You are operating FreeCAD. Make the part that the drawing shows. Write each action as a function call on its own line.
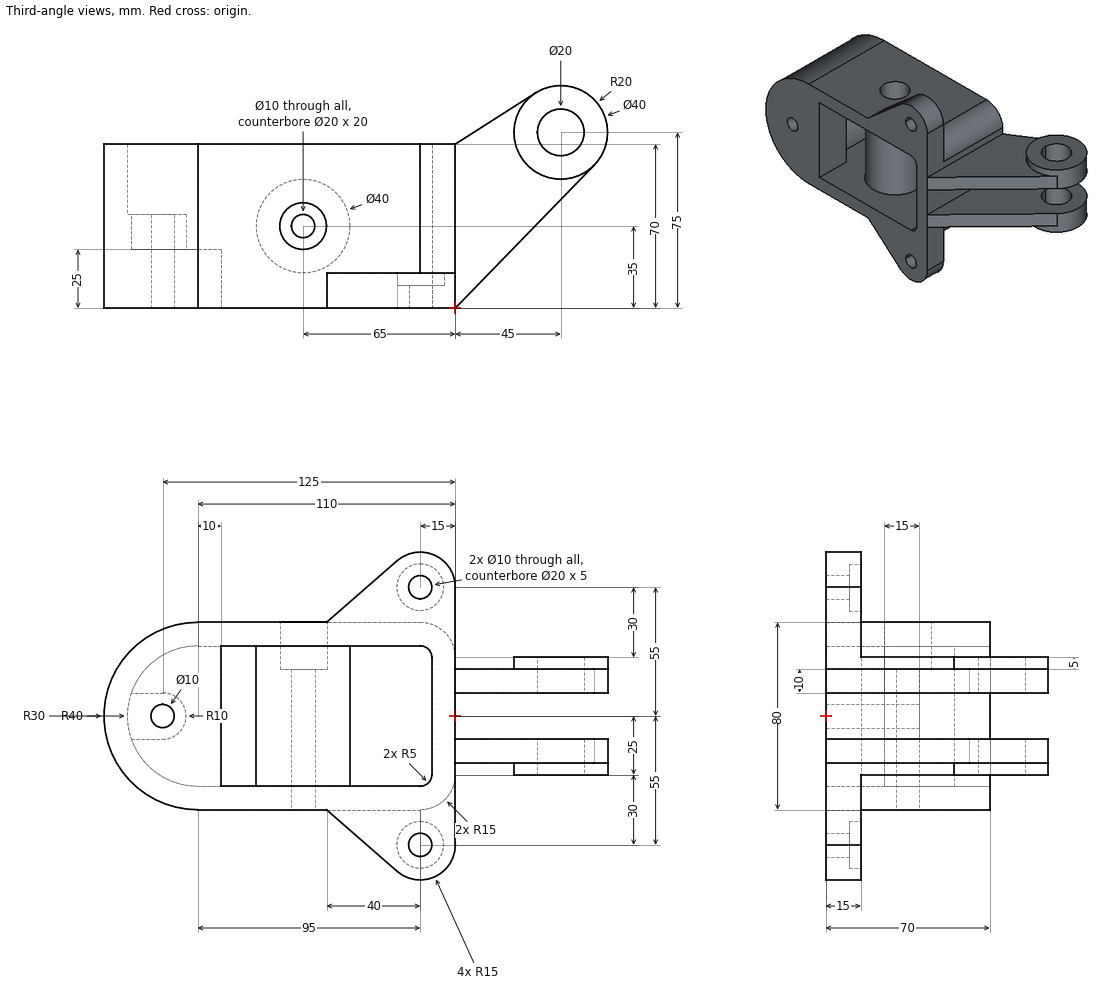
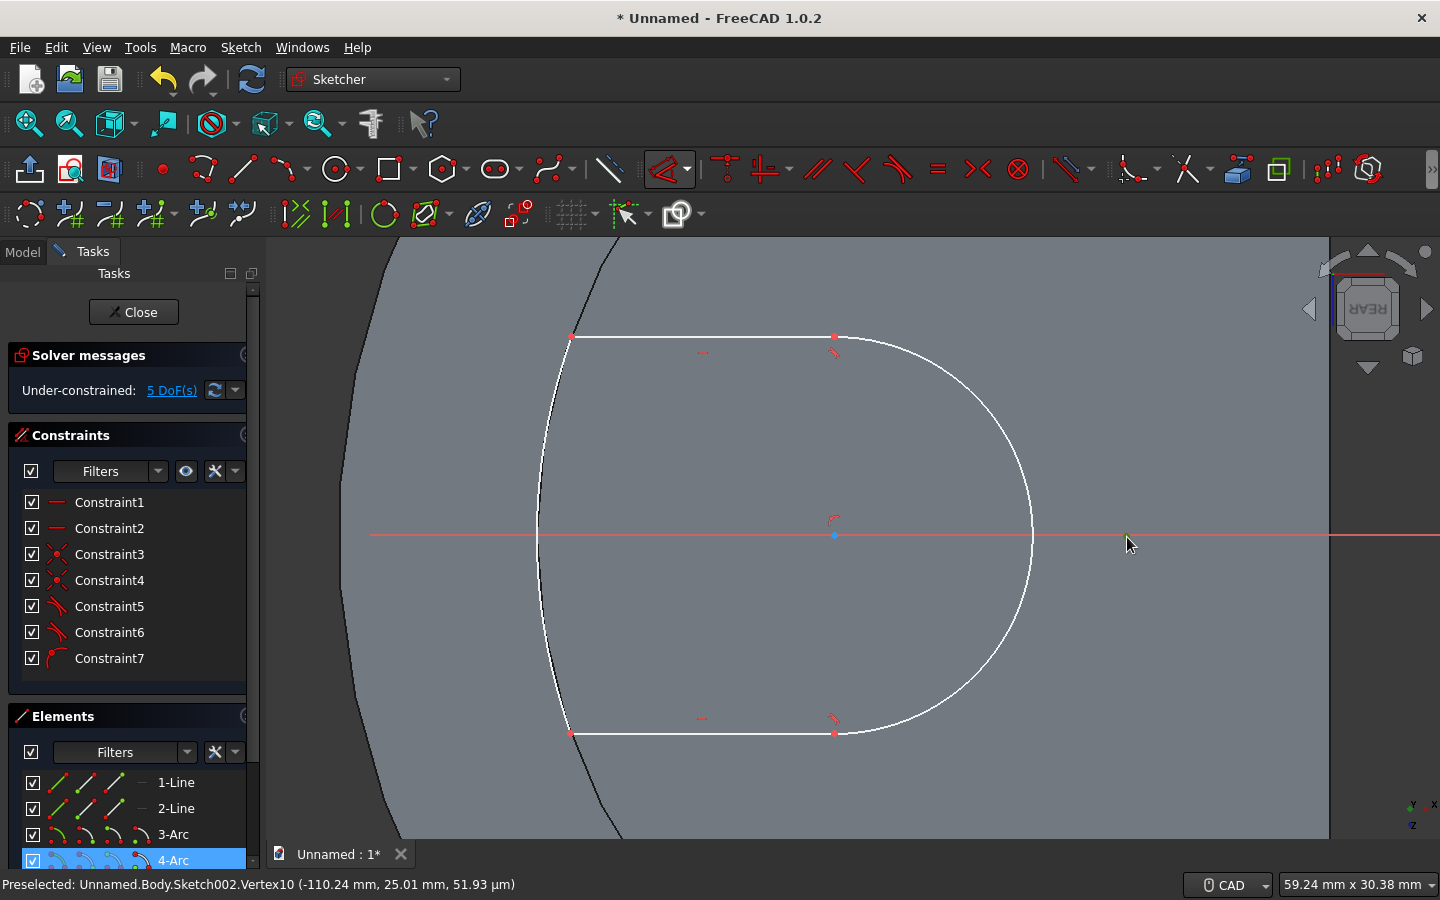
click(434, 535)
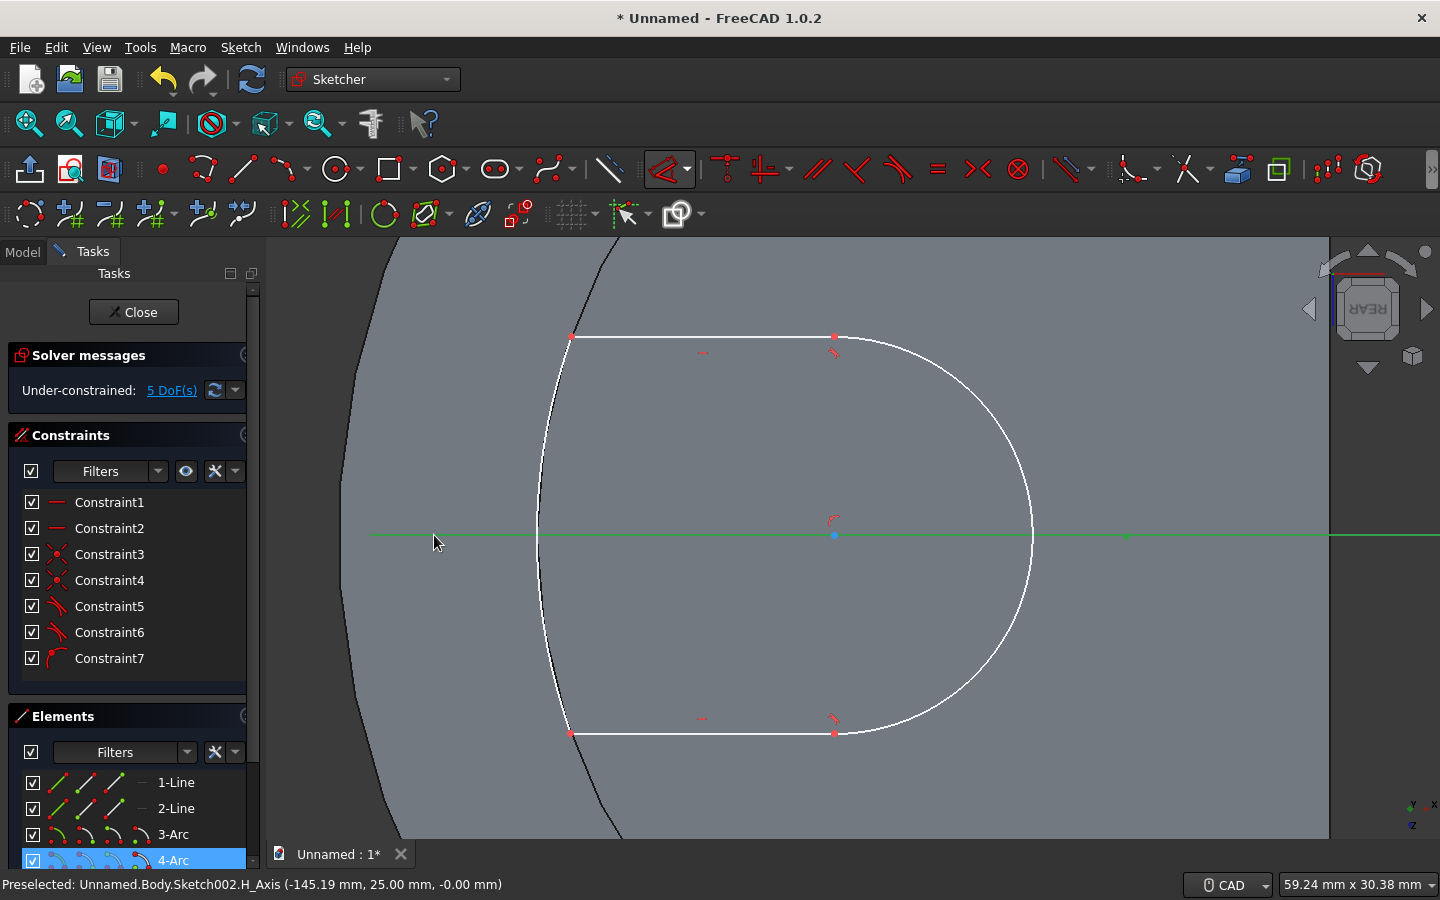
key(c)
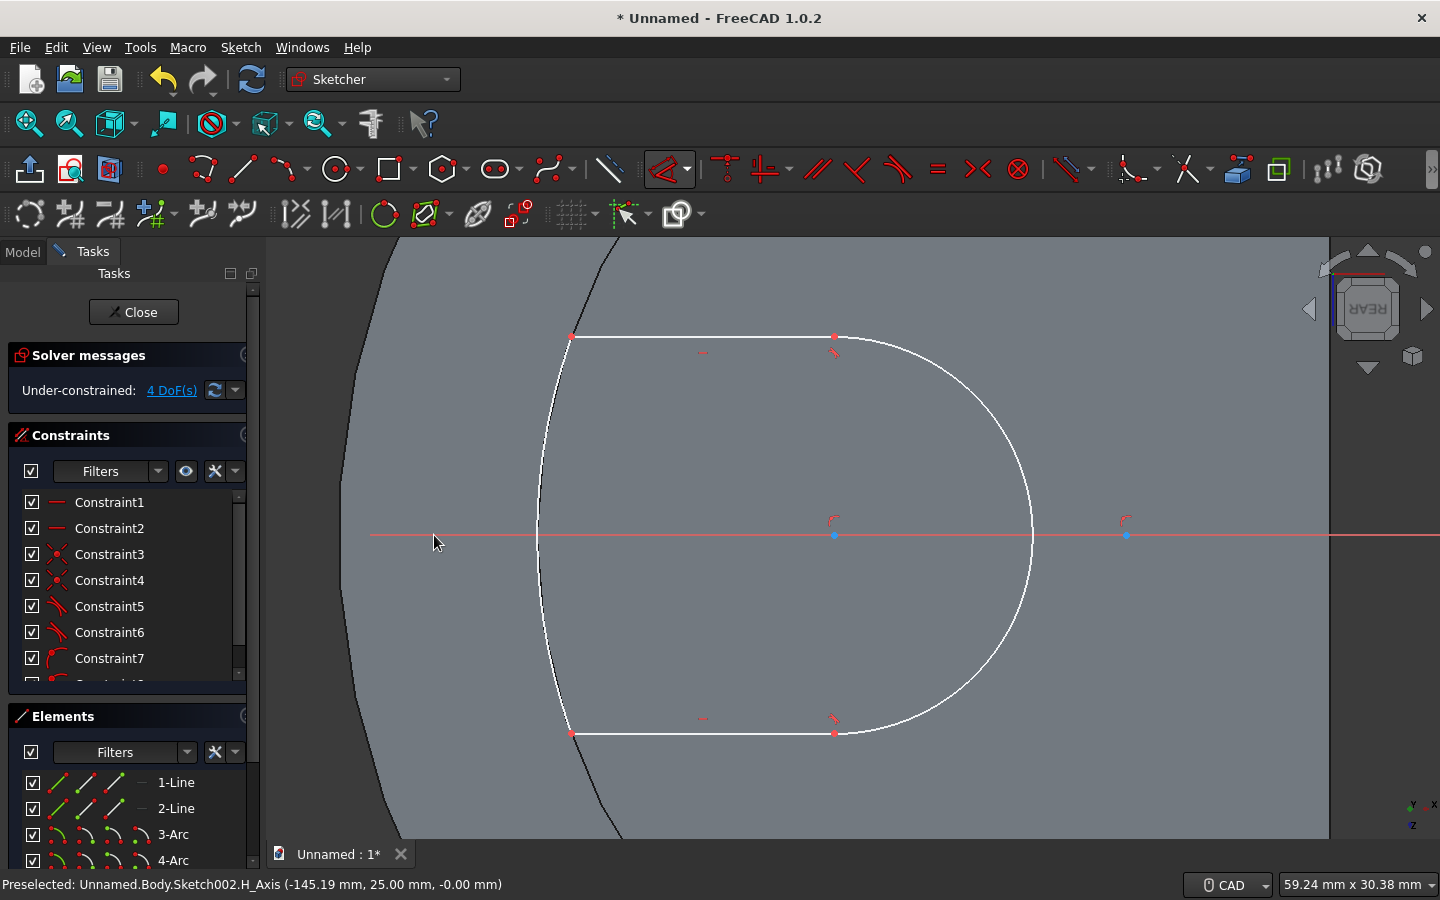
click(995, 652)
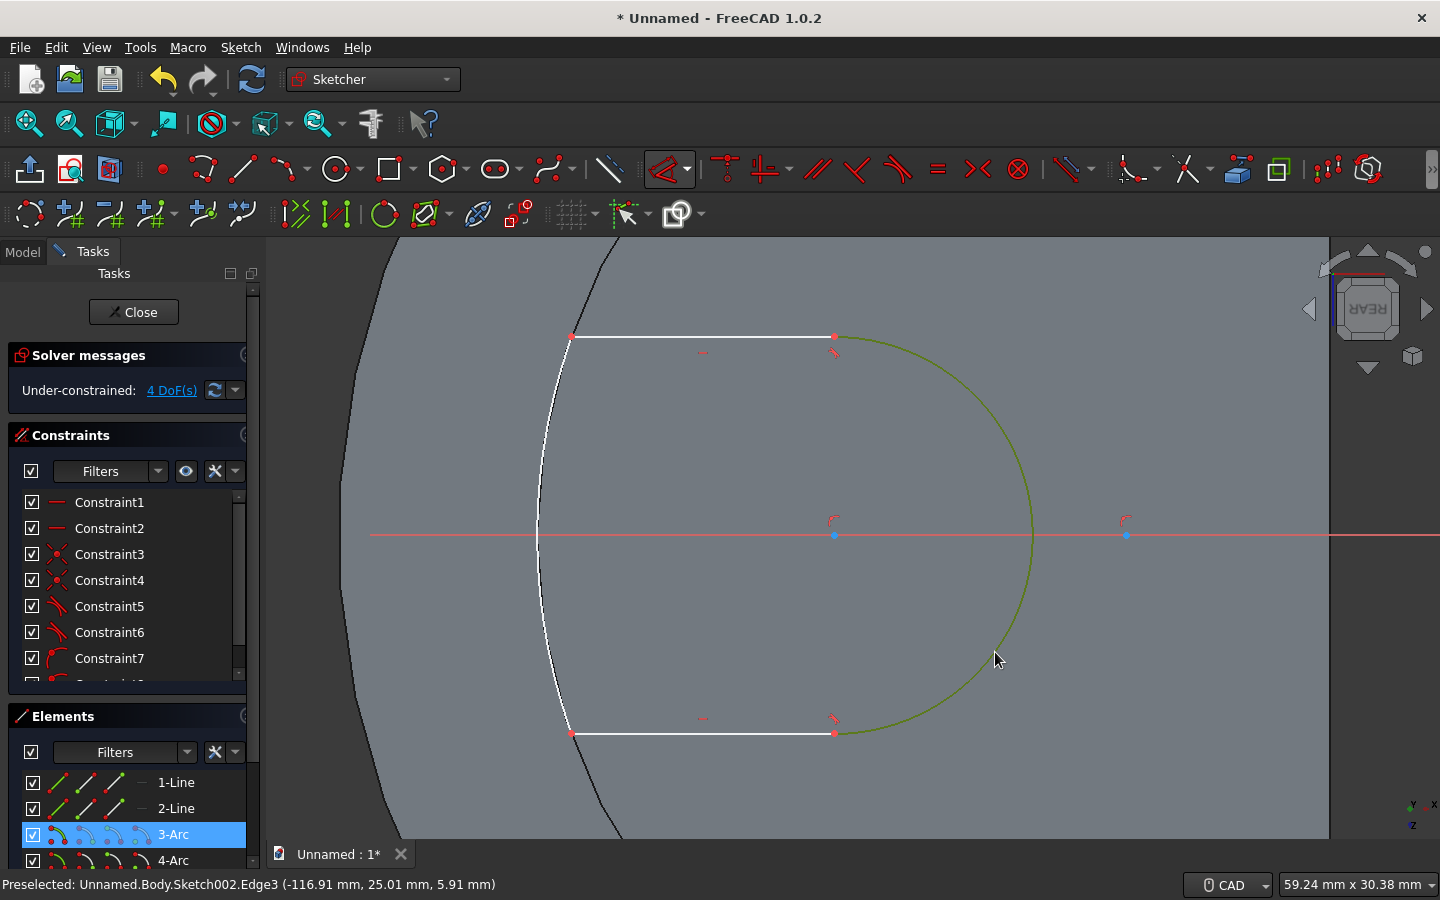
key(k)
key(r)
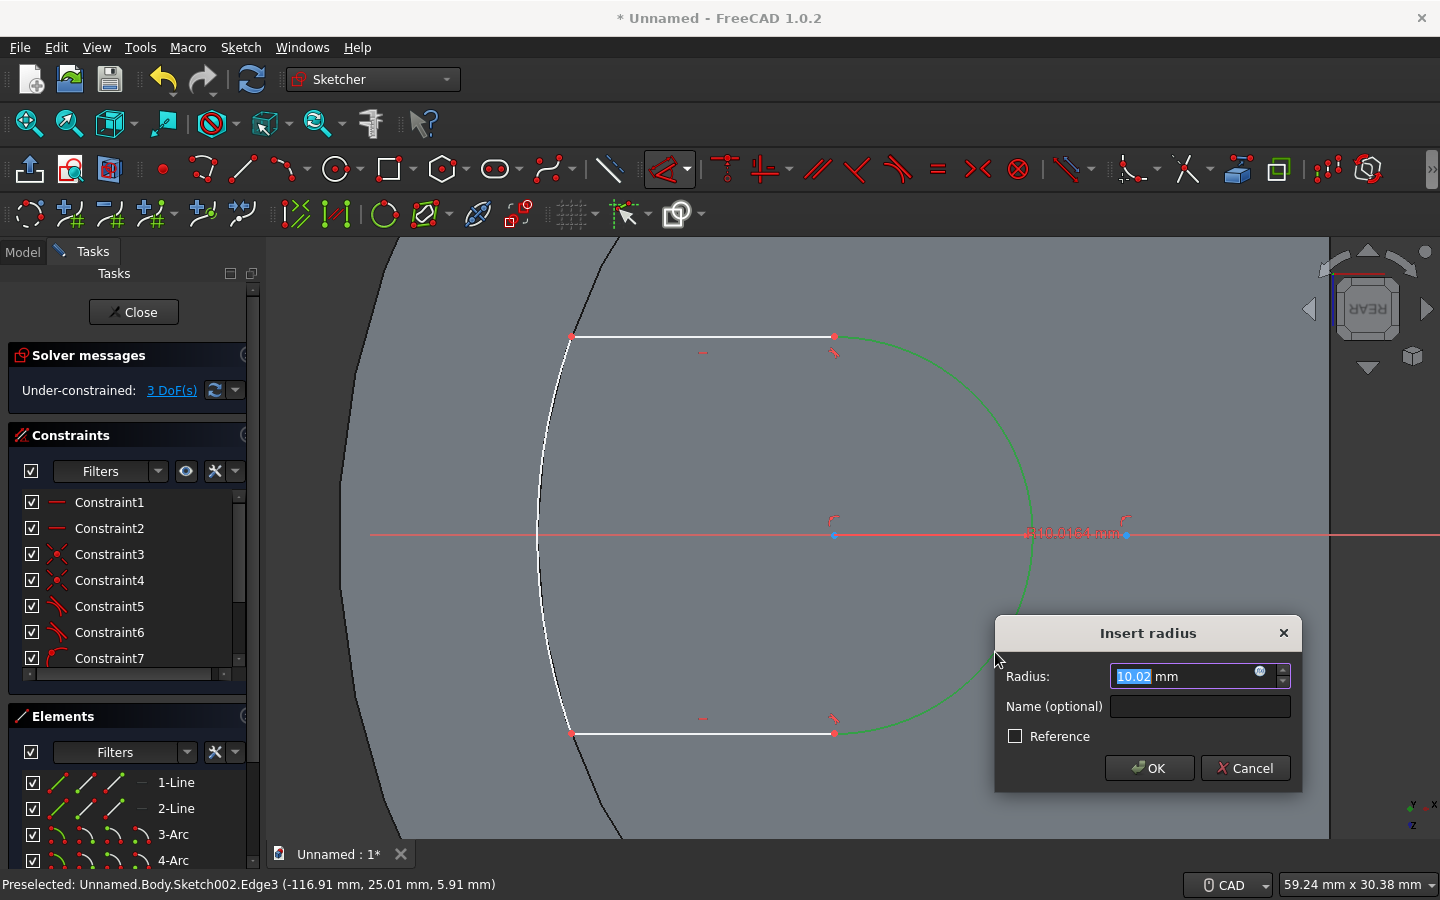
text(10)
key(Return)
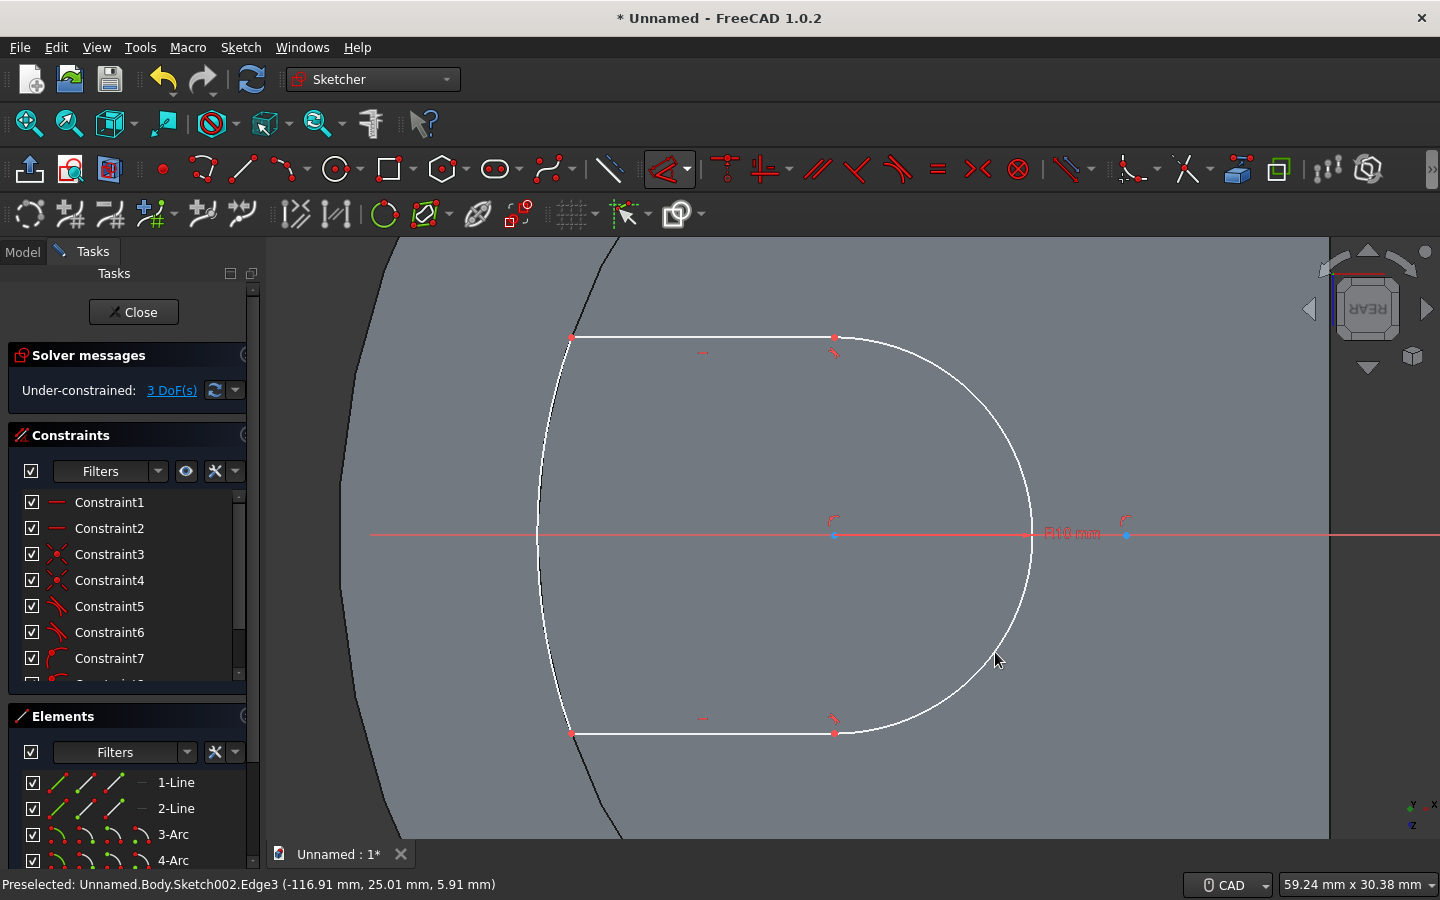
click(543, 455)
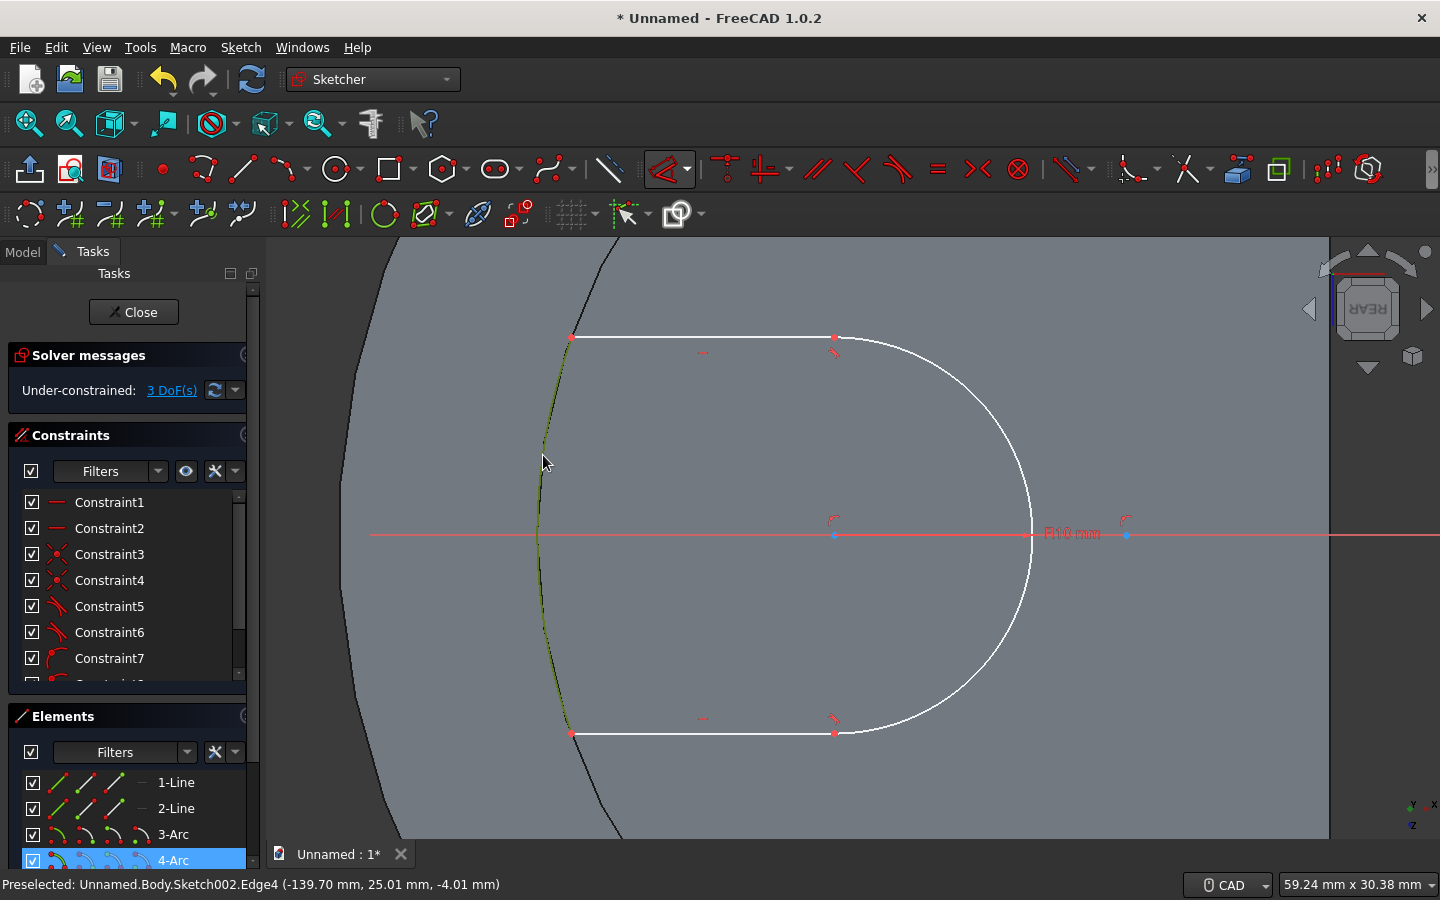
click(690, 170)